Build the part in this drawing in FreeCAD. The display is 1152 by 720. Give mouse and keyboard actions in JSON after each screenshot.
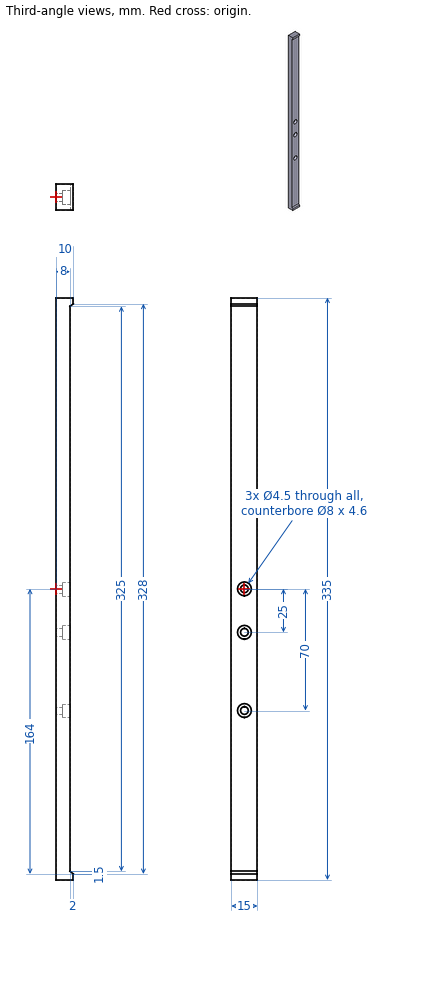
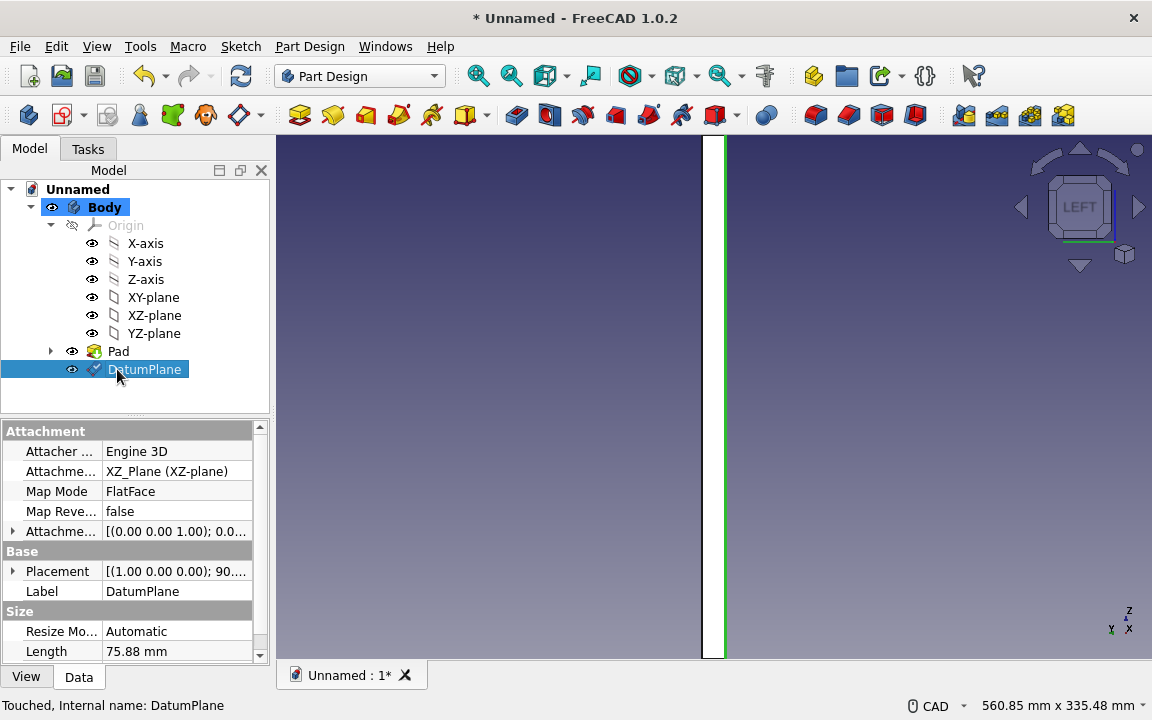
{"action": "left_click", "coordinate": [62, 116]}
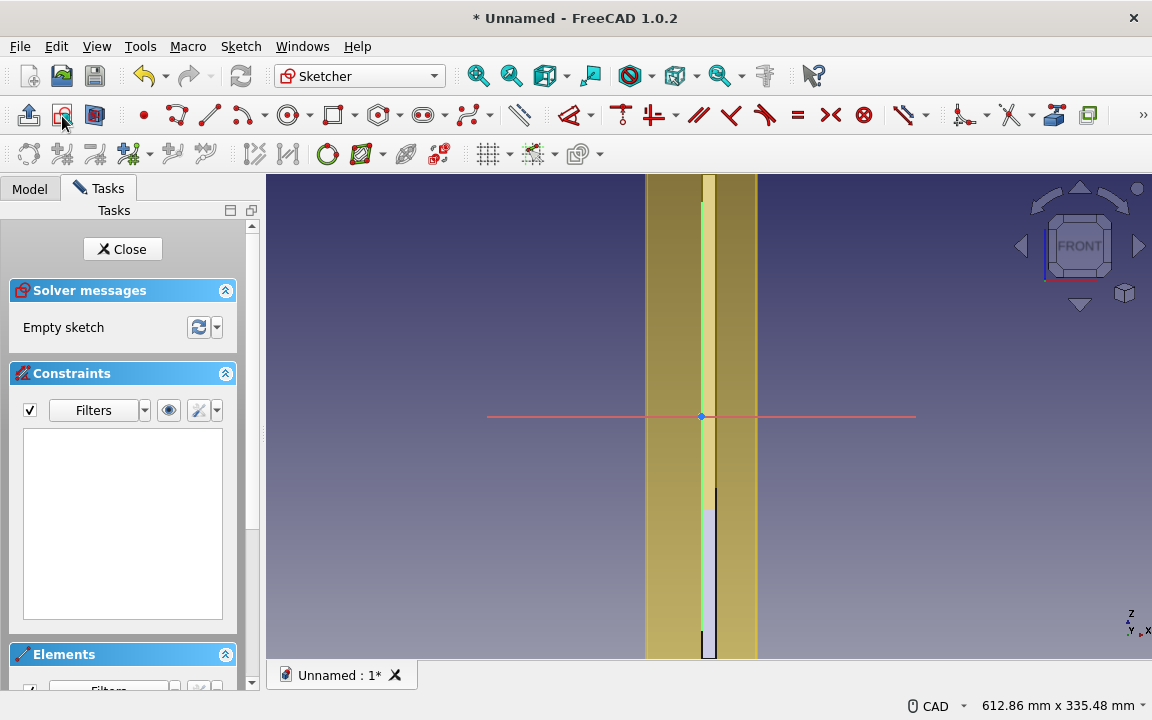
{"action": "scroll", "coordinate": [501, 416], "scroll_direction": "down", "scroll_amount": 2}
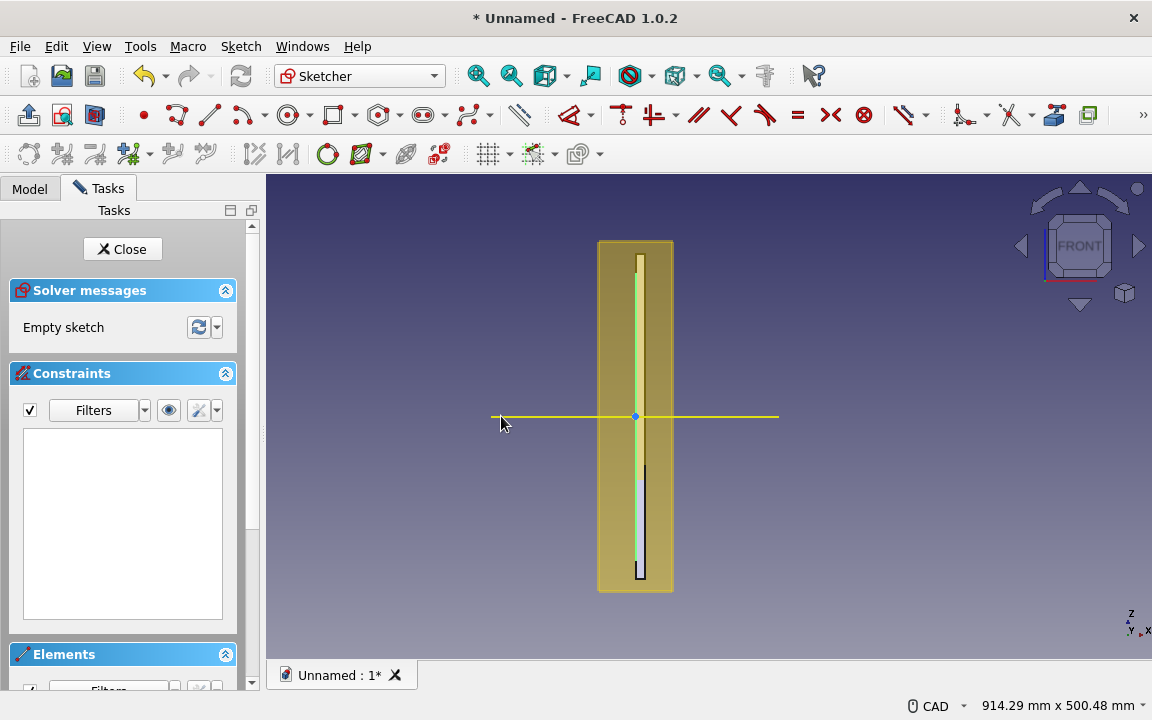
{"action": "left_click", "coordinate": [177, 116]}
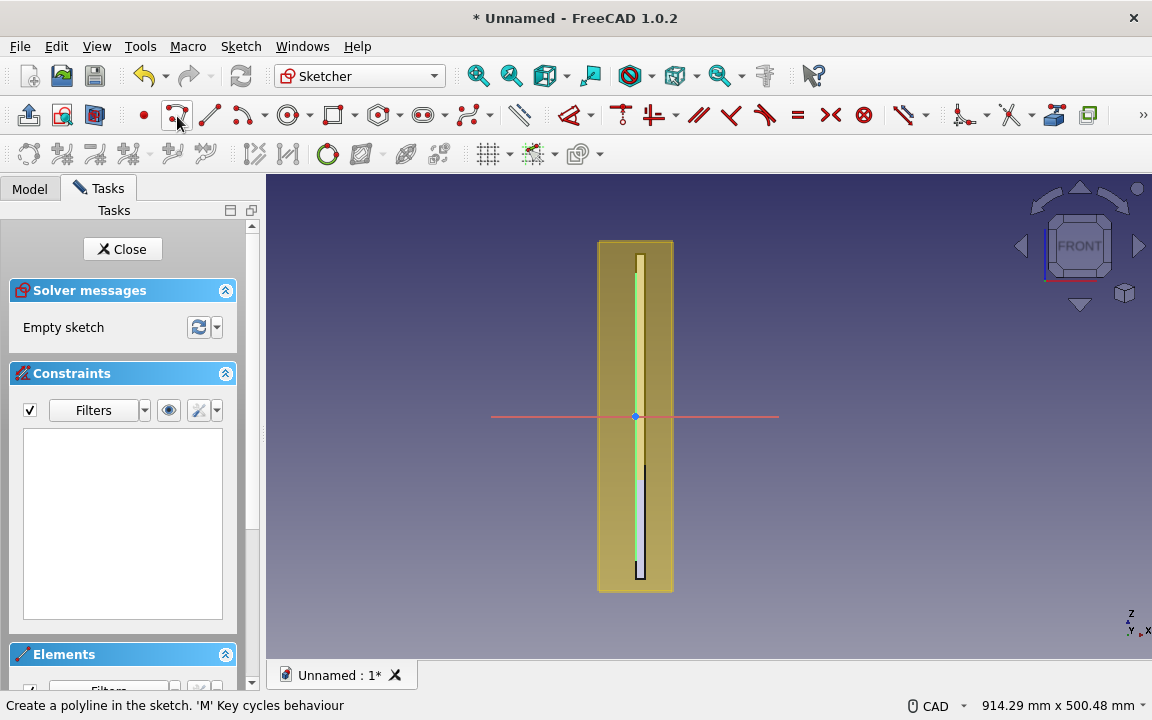
{"action": "scroll", "coordinate": [643, 259], "scroll_direction": "up", "scroll_amount": 4}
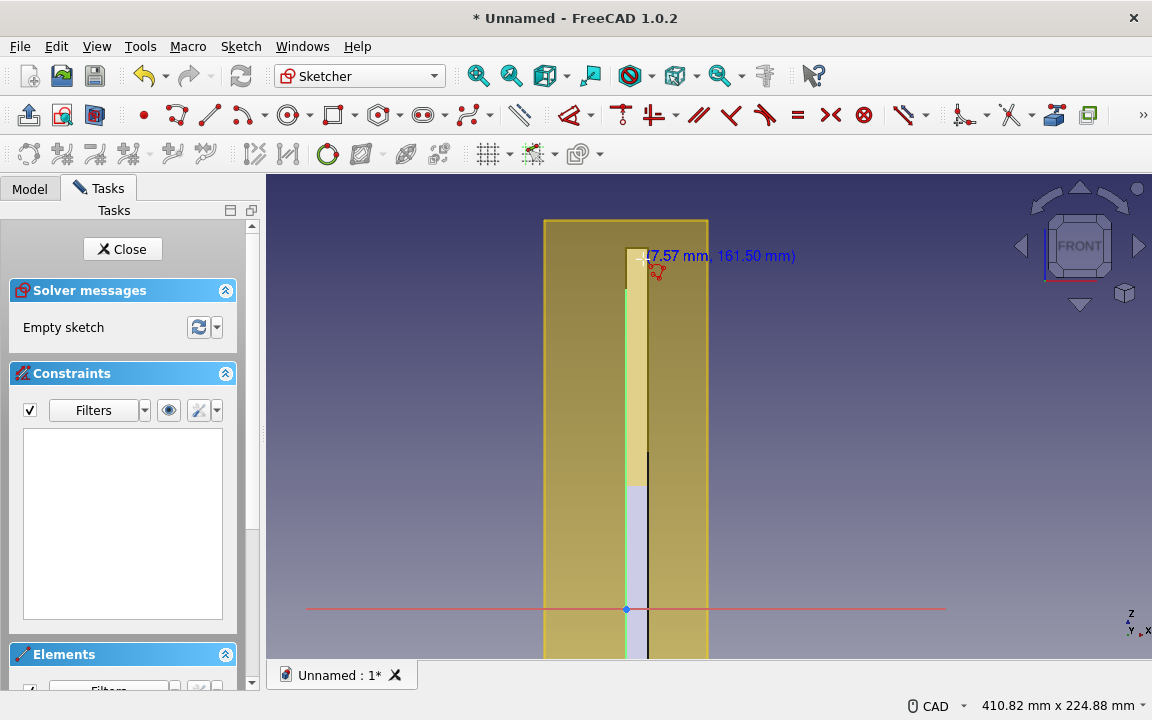
{"action": "left_click", "coordinate": [643, 259]}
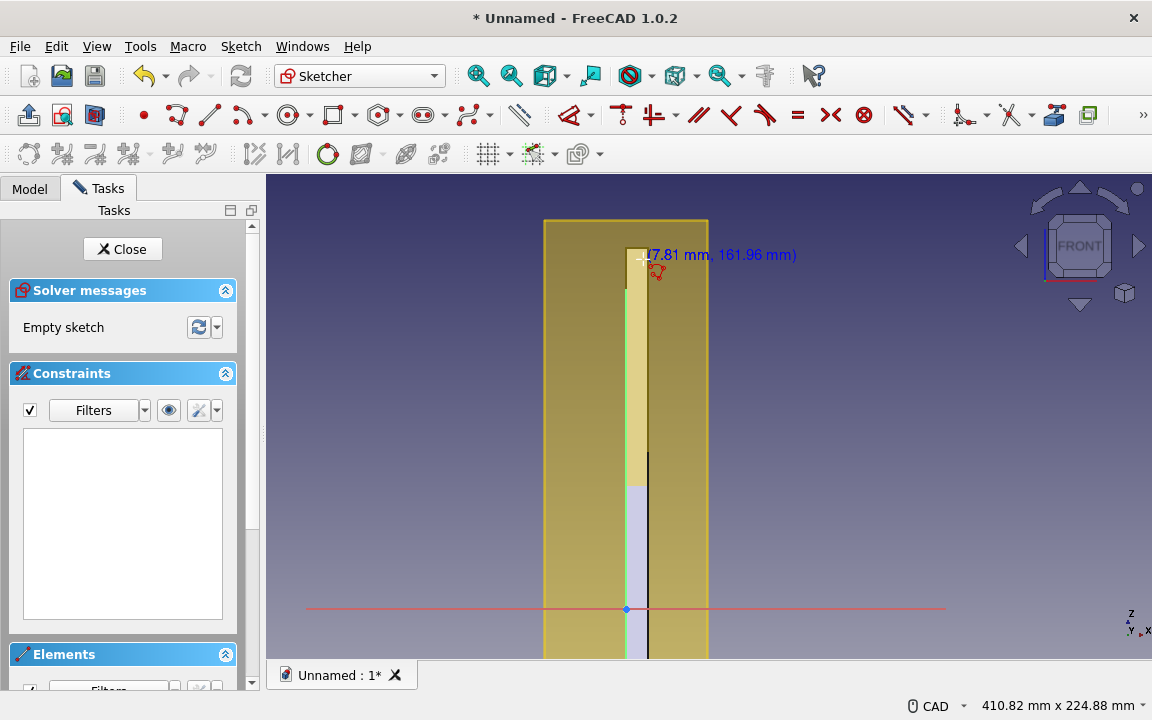
{"action": "scroll", "coordinate": [643, 259], "scroll_direction": "down", "scroll_amount": 4}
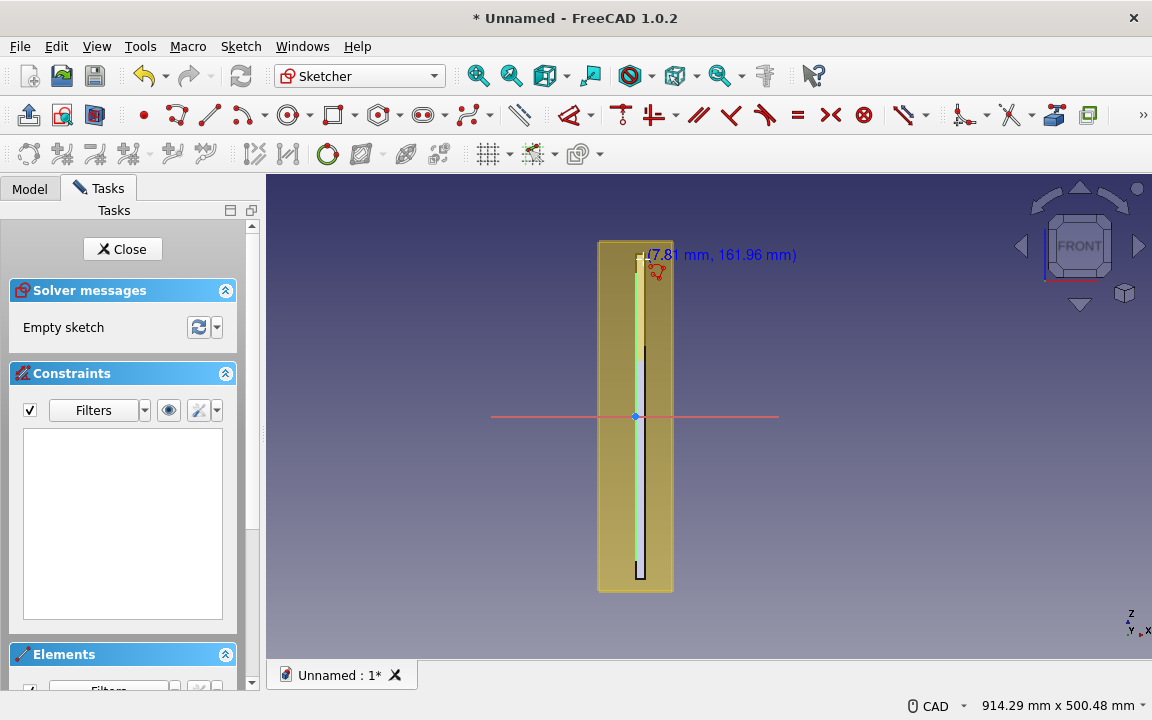
{"action": "scroll", "coordinate": [643, 574], "scroll_direction": "up", "scroll_amount": 4}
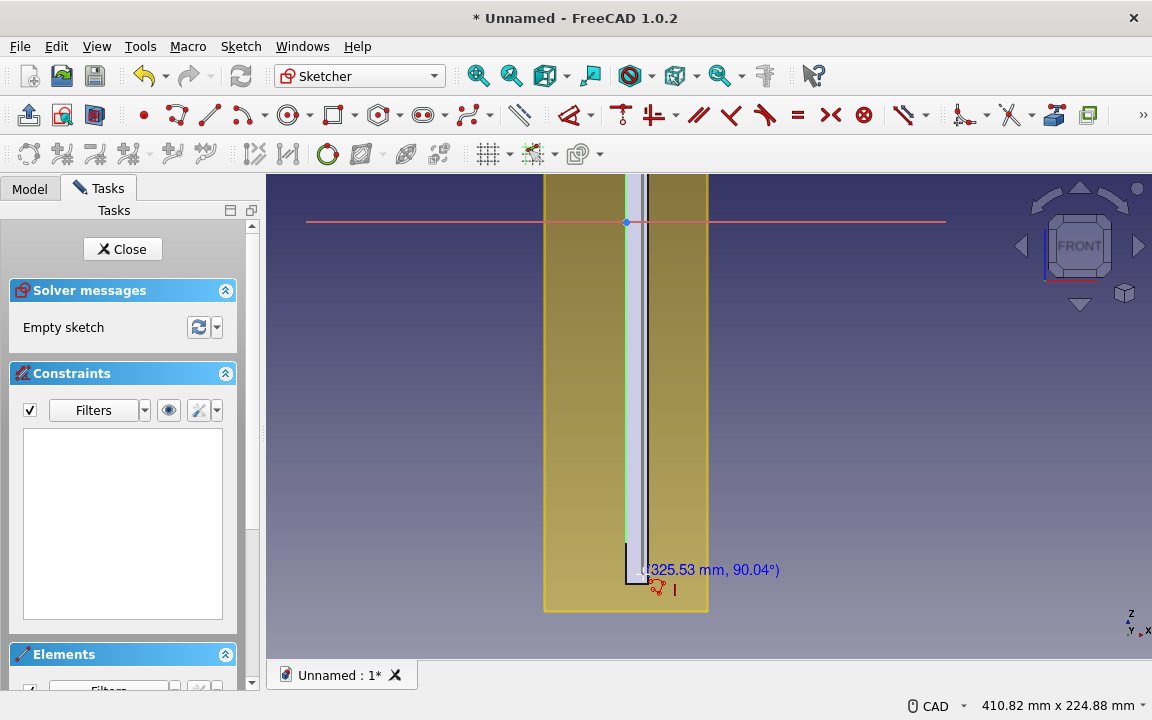
{"action": "left_click", "coordinate": [643, 573]}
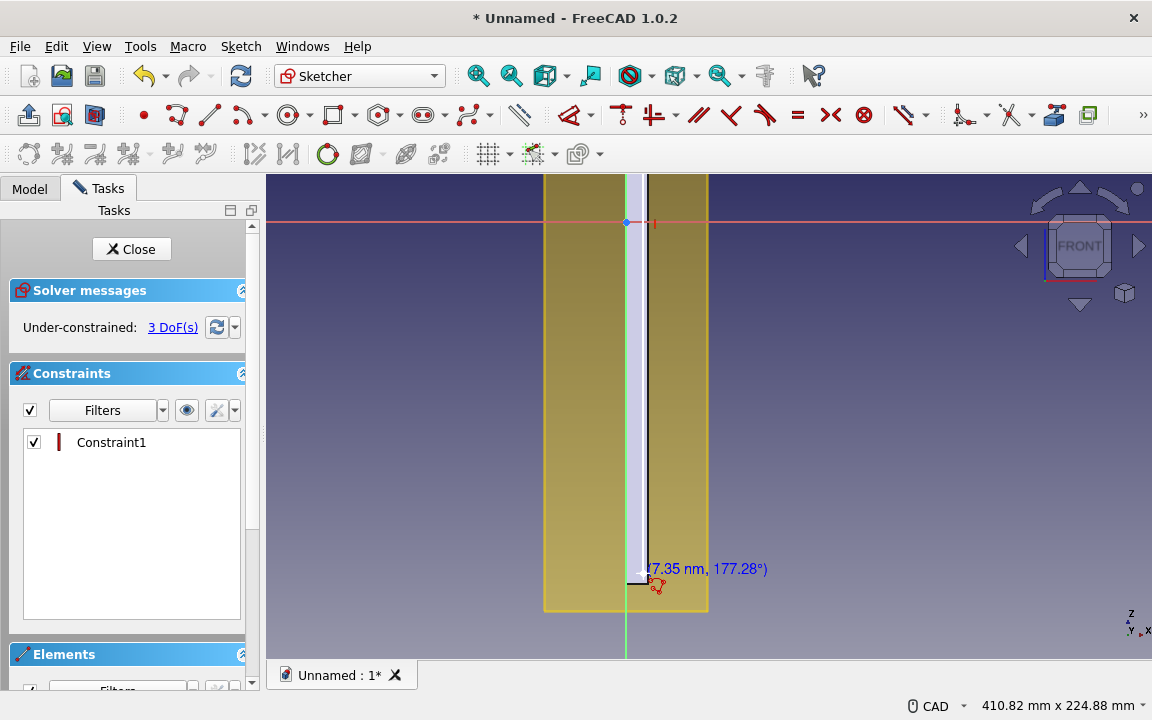
{"action": "scroll", "coordinate": [648, 576], "scroll_direction": "up", "scroll_amount": 6}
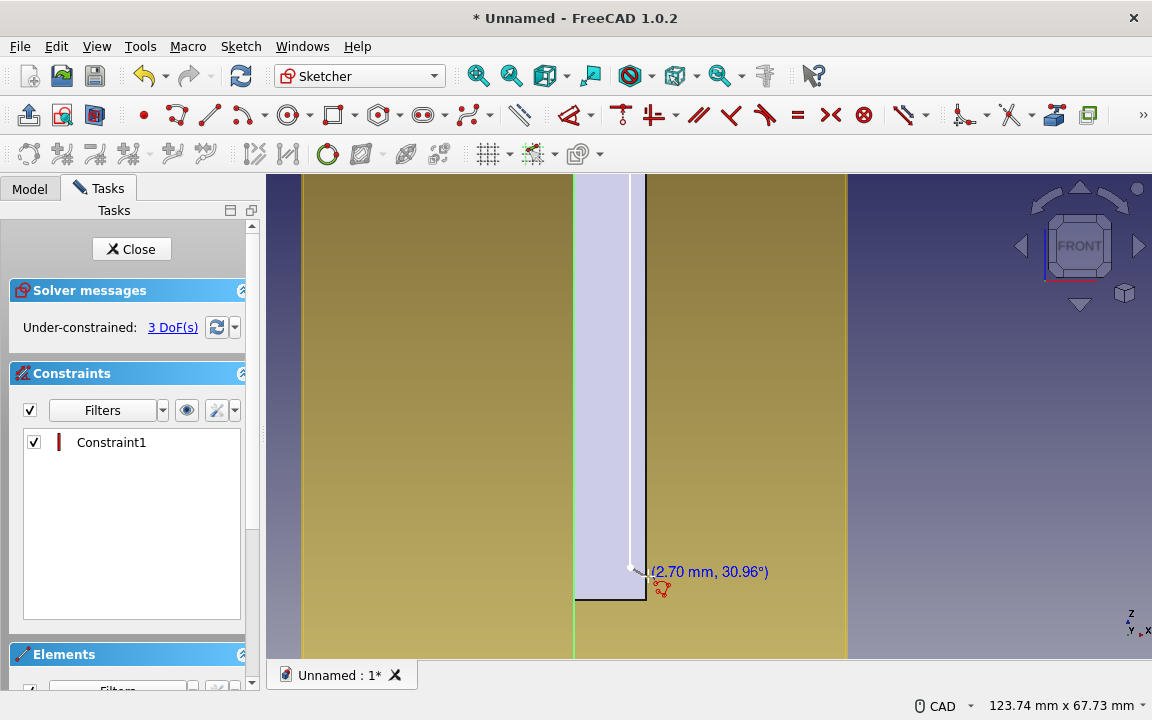
{"action": "left_click", "coordinate": [646, 575]}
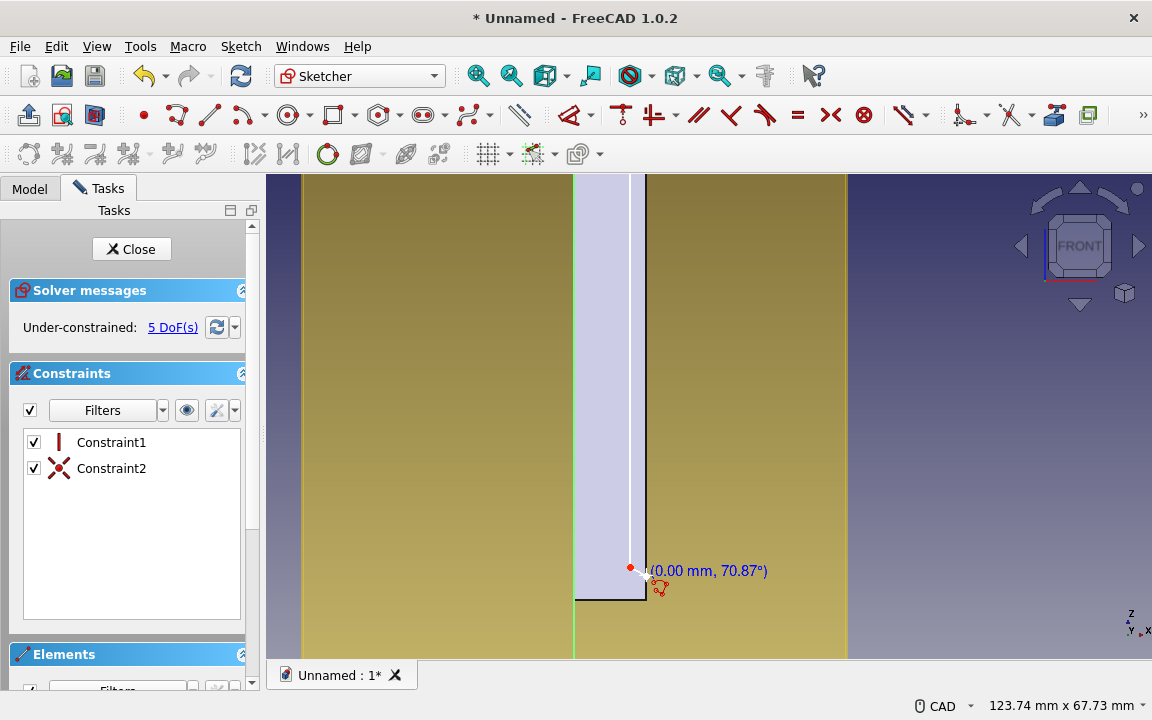
{"action": "scroll", "coordinate": [645, 576], "scroll_direction": "down", "scroll_amount": 10}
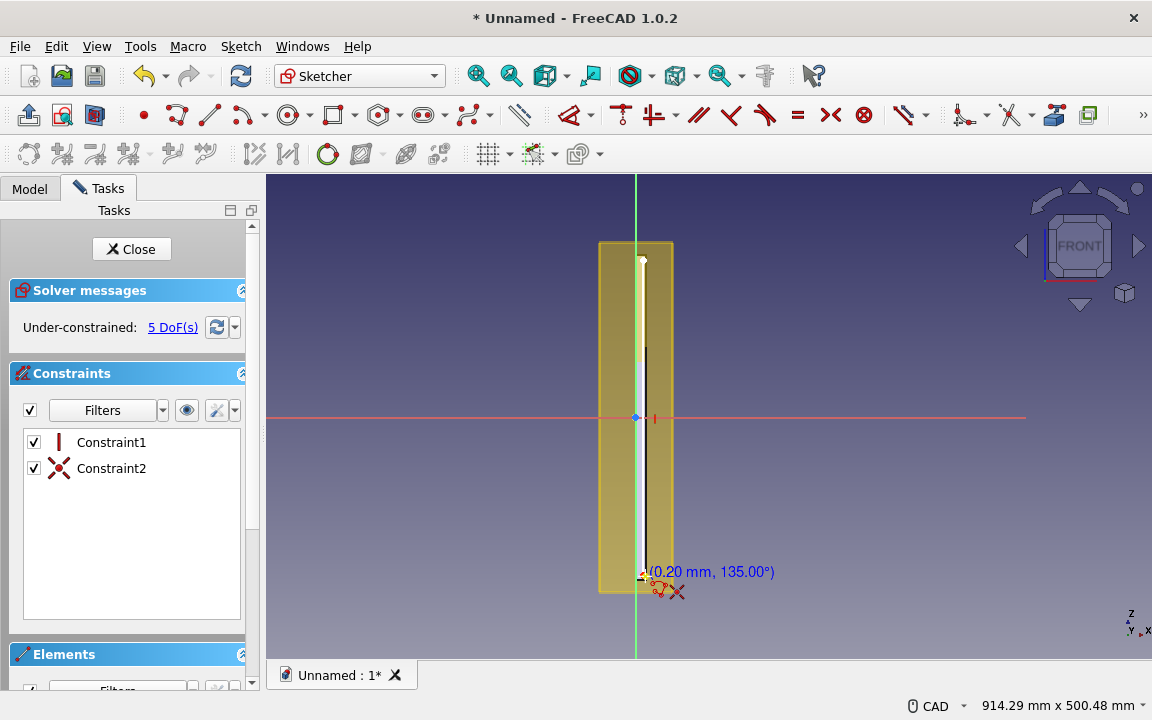
{"action": "scroll", "coordinate": [646, 259], "scroll_direction": "up", "scroll_amount": 10}